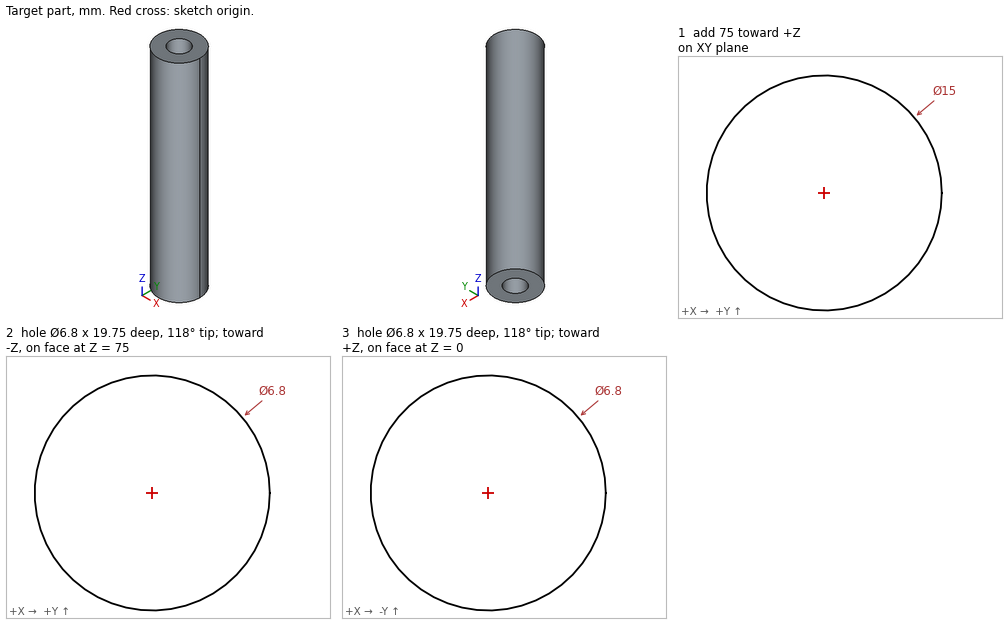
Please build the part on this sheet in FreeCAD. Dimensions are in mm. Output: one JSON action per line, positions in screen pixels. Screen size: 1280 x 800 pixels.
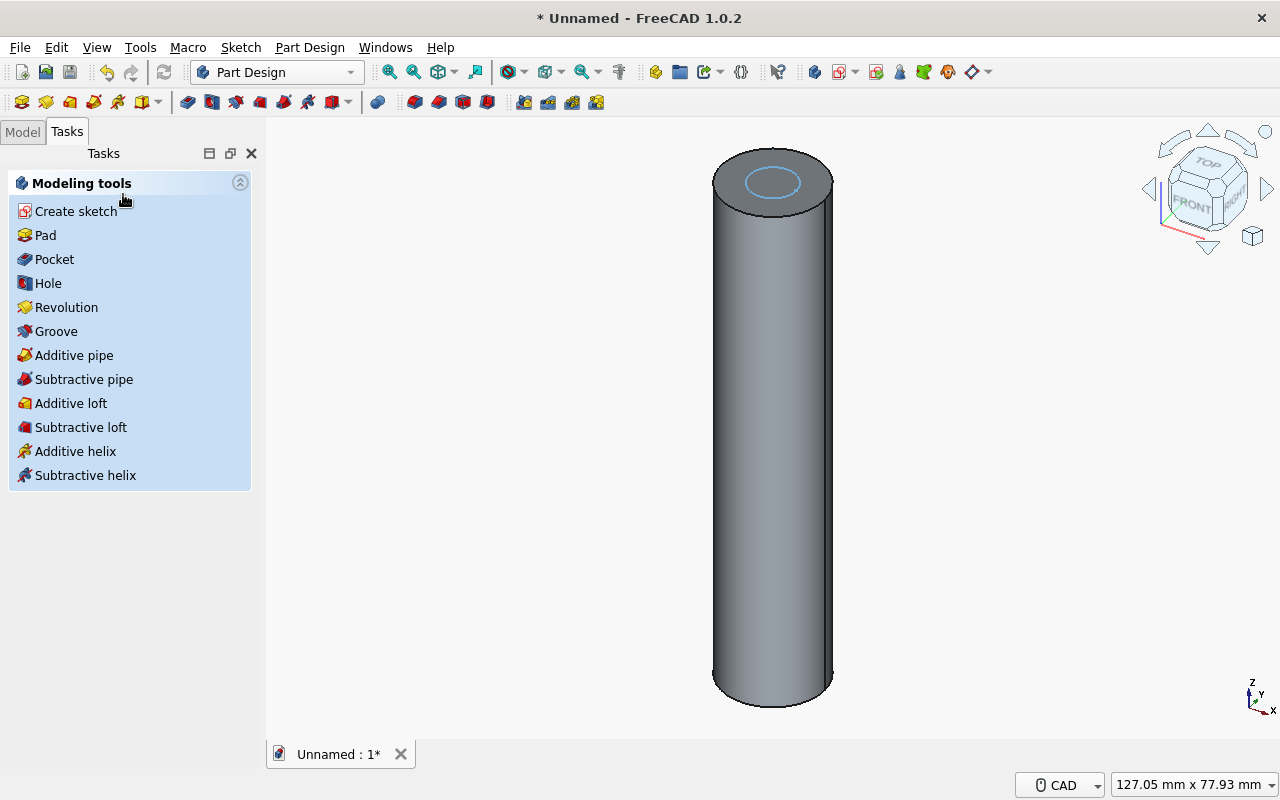
{"action": "left_click", "coordinate": [212, 102]}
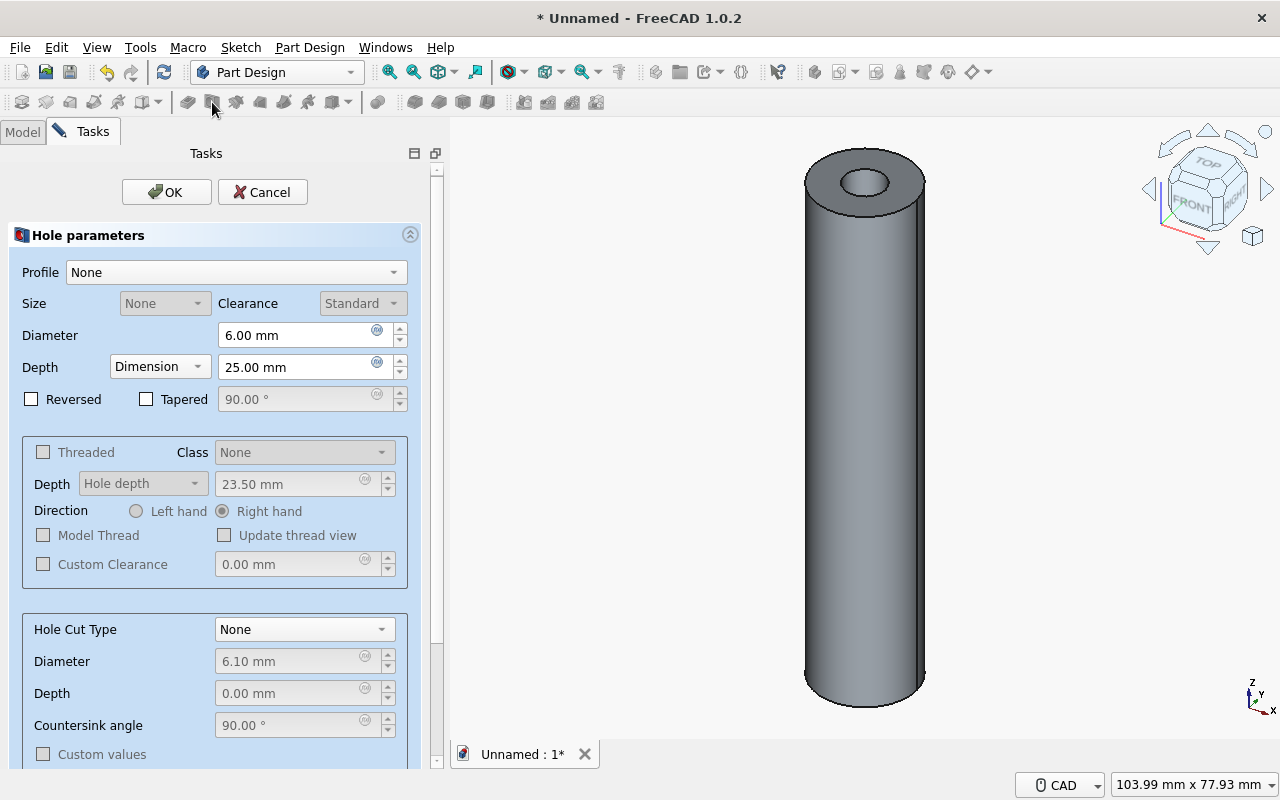
{"action": "triple_click", "coordinate": [305, 335]}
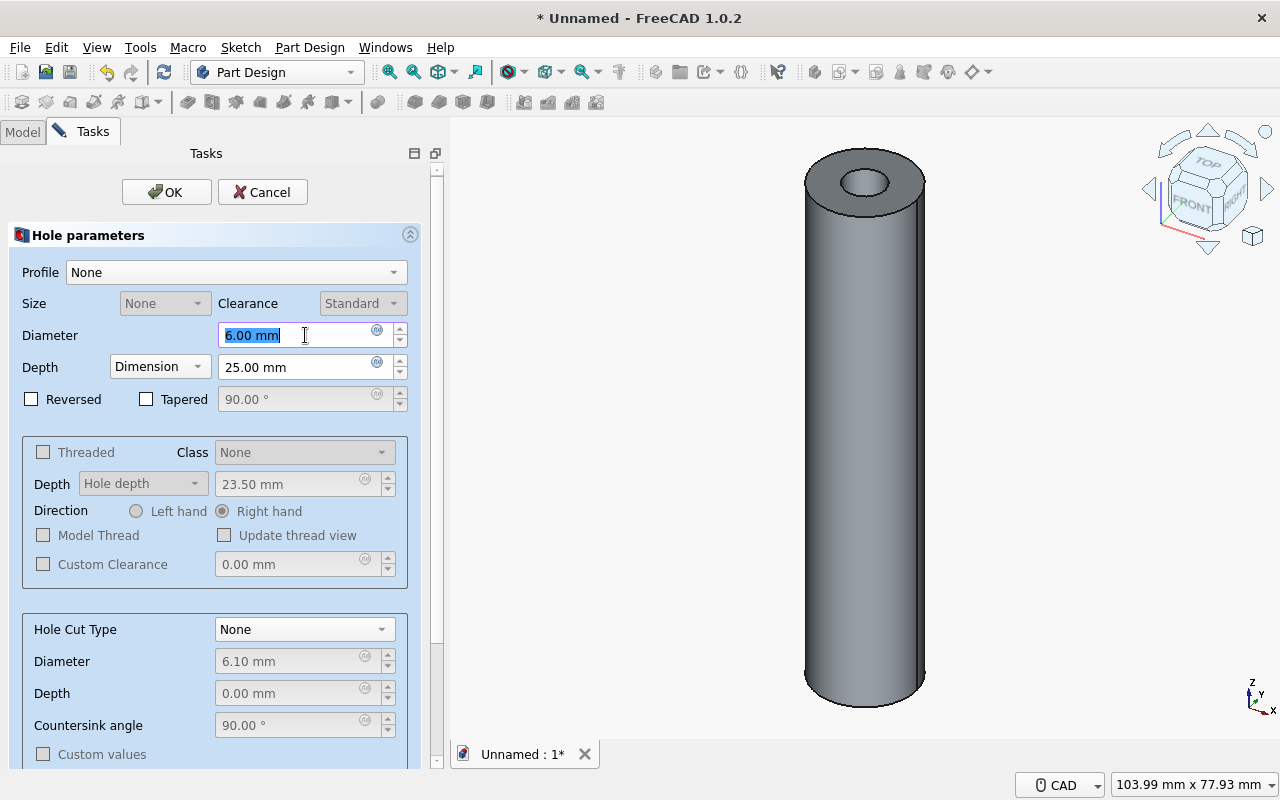
{"action": "type", "text": "6.8"}
{"action": "key", "text": "Tab"}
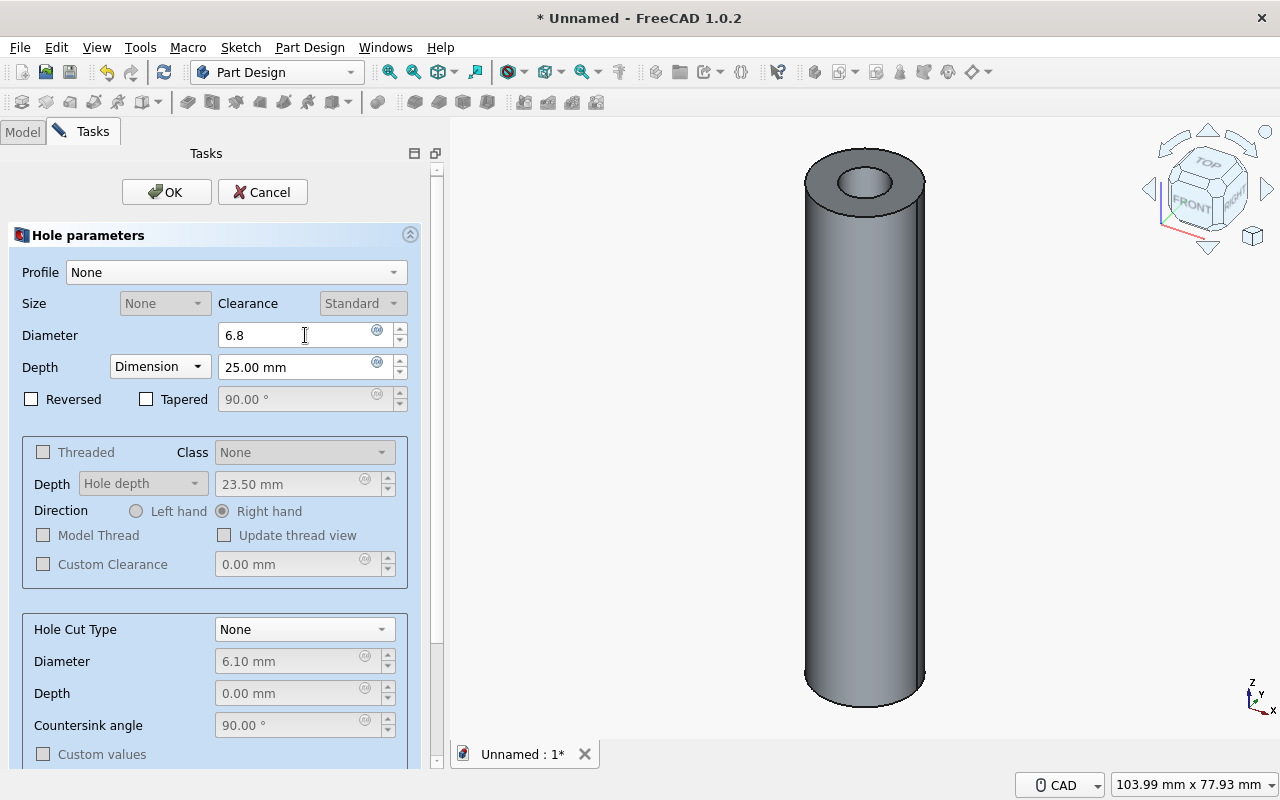
{"action": "triple_click", "coordinate": [305, 367]}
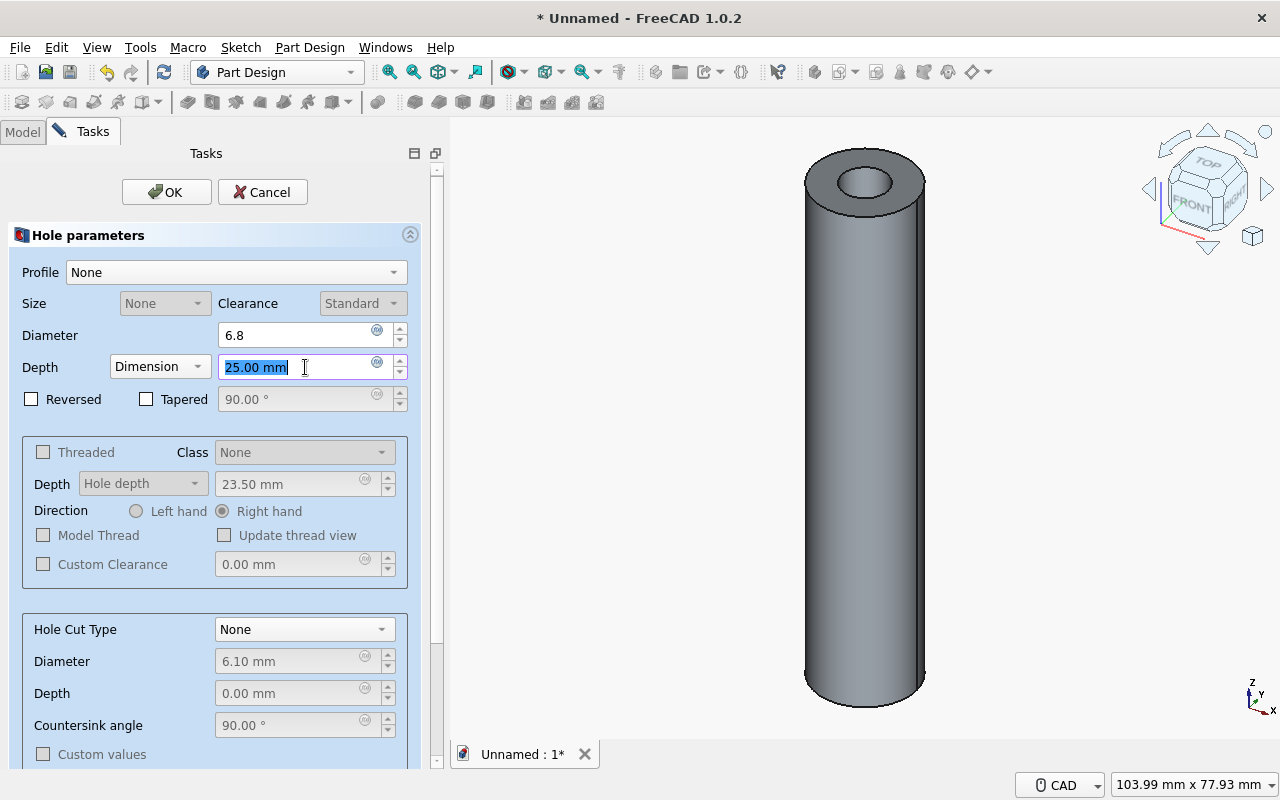
{"action": "type", "text": "19.75"}
{"action": "key", "text": "Tab"}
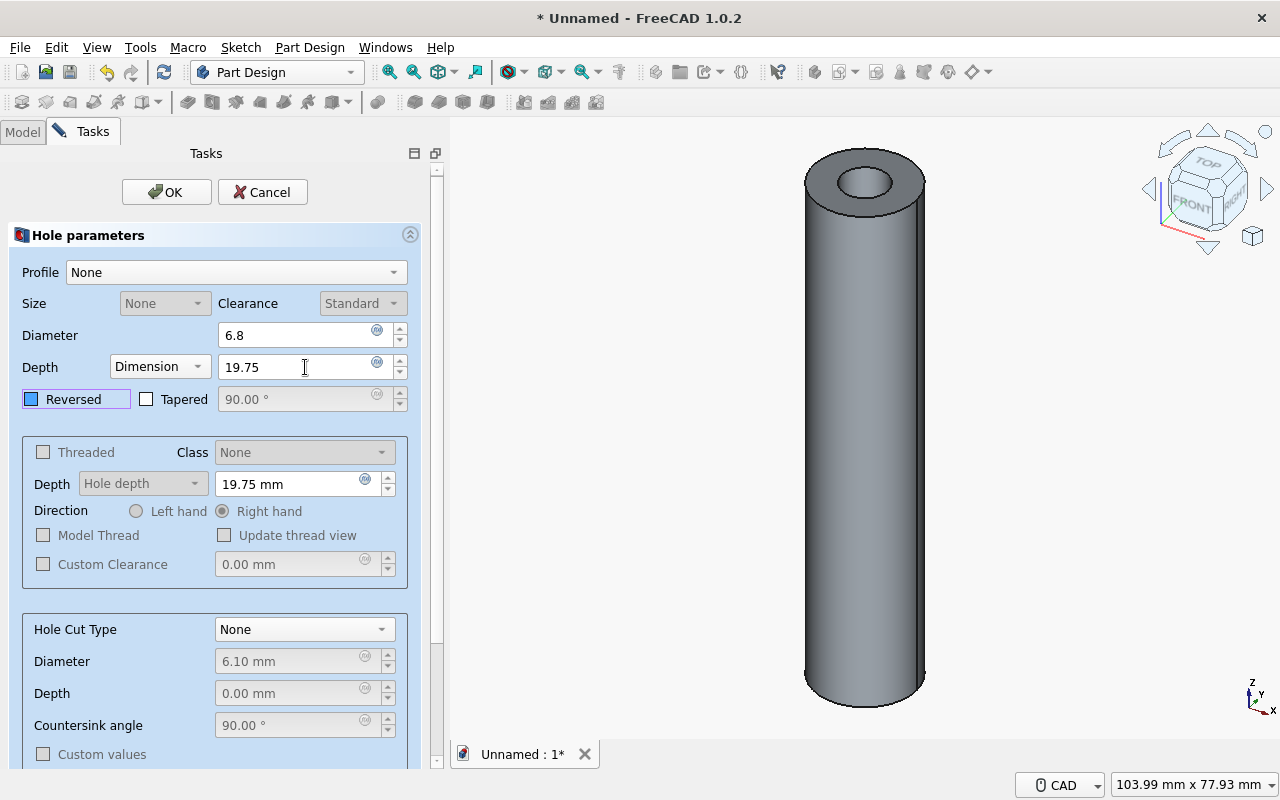
{"action": "left_click", "coordinate": [167, 192]}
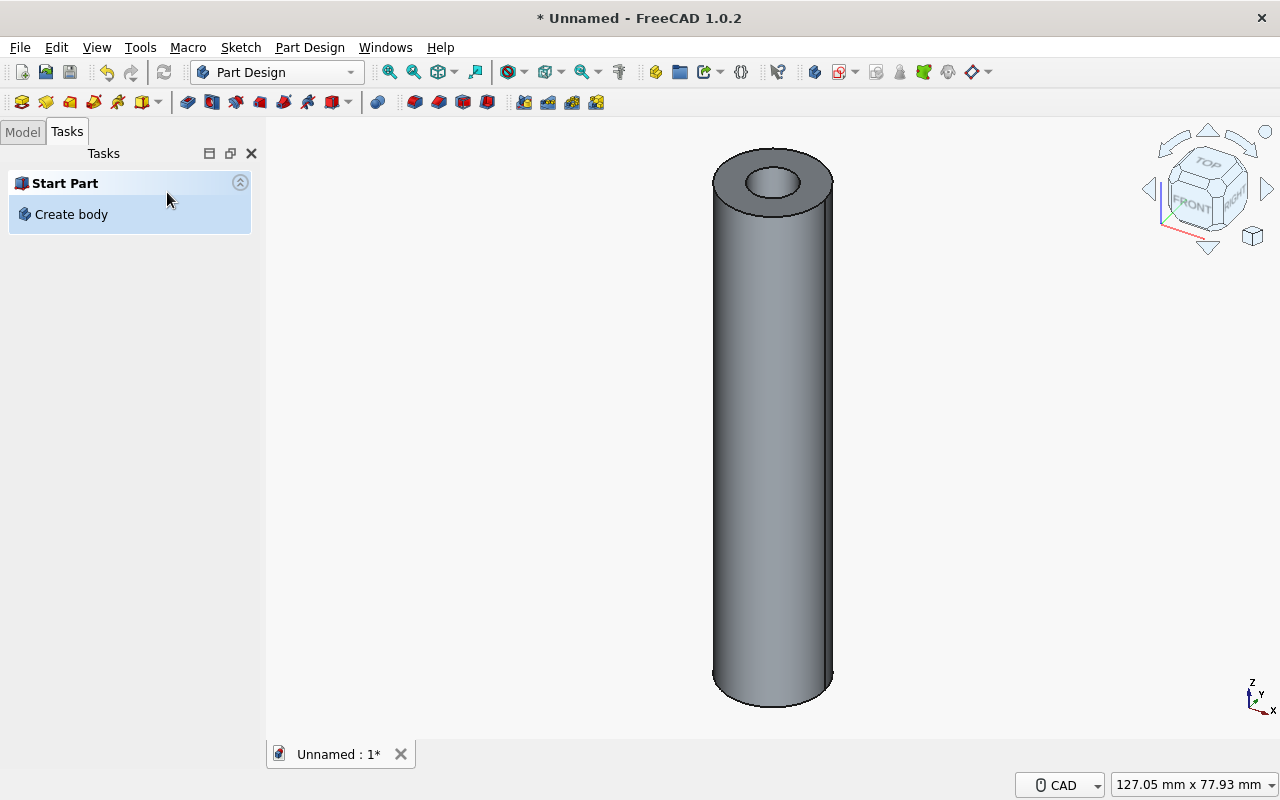
{"action": "key", "text": "5"}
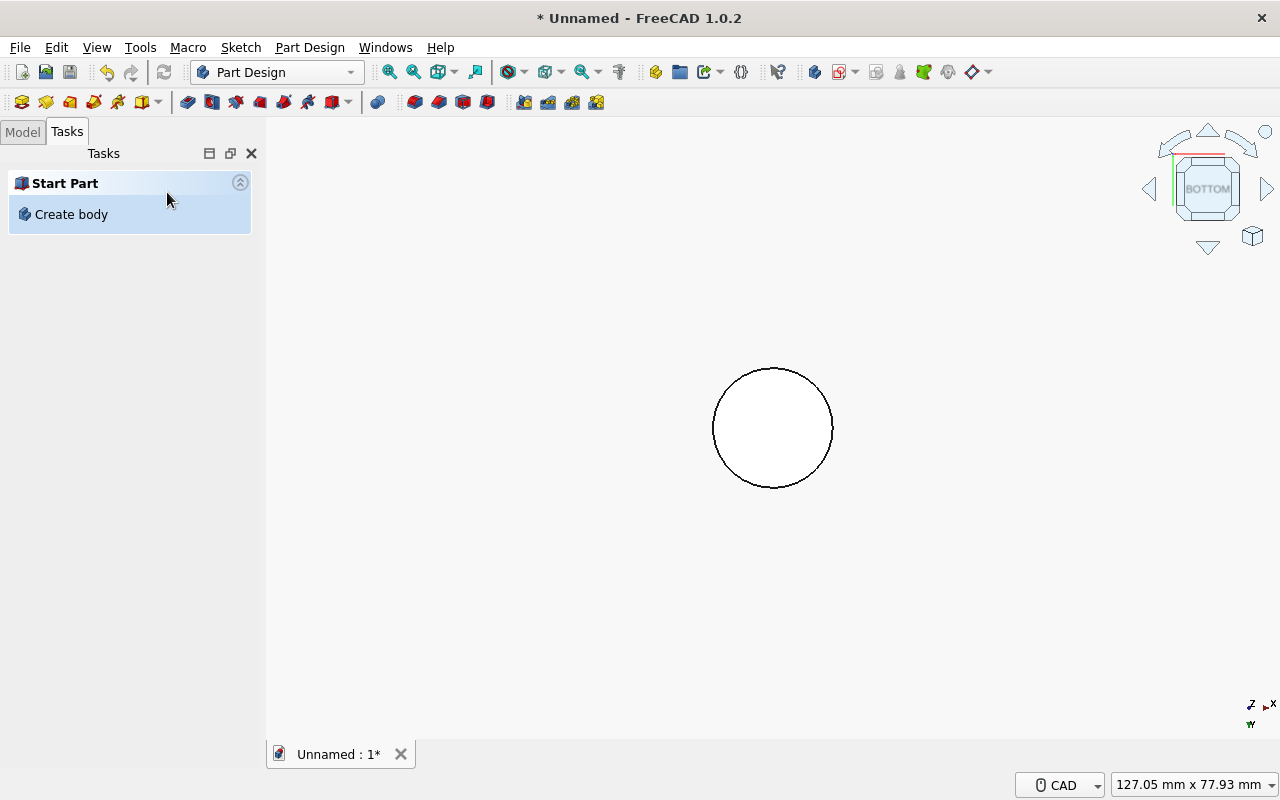
{"action": "left_click", "coordinate": [390, 72]}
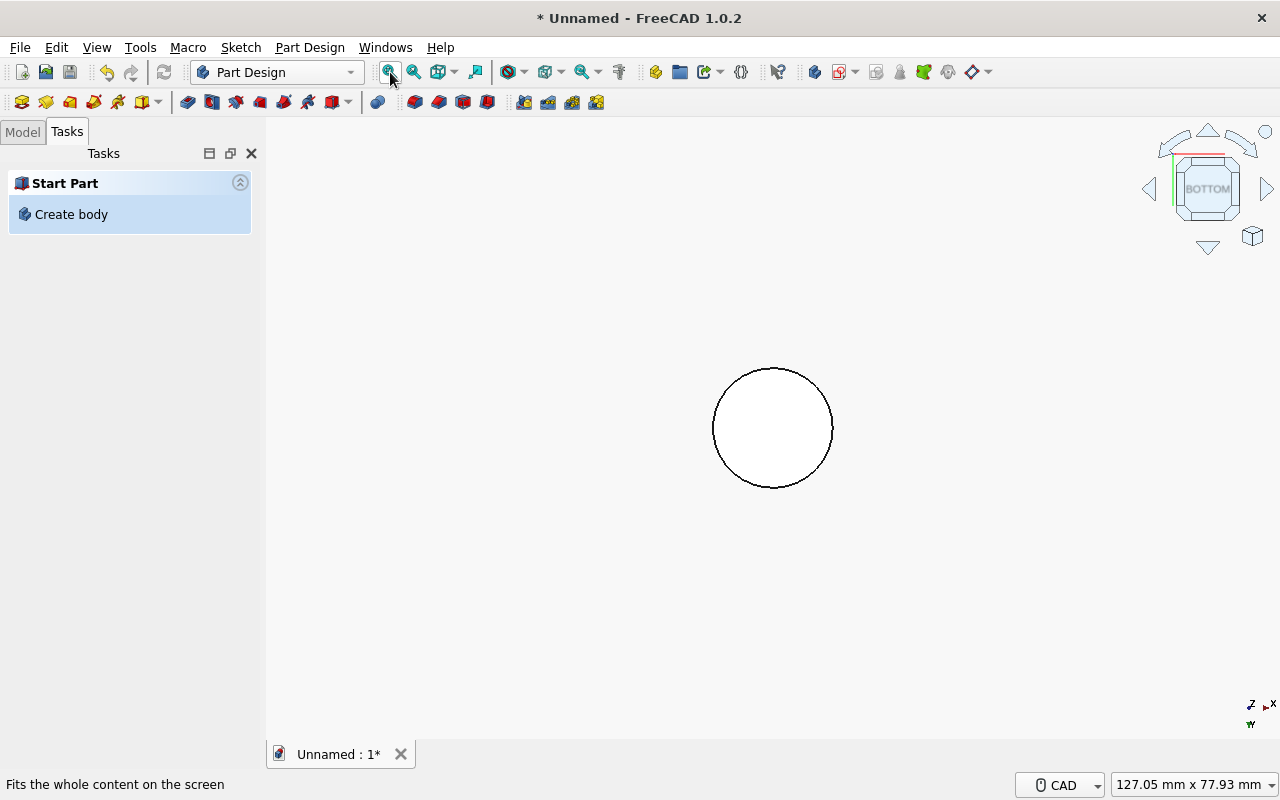
{"action": "left_click", "coordinate": [773, 427]}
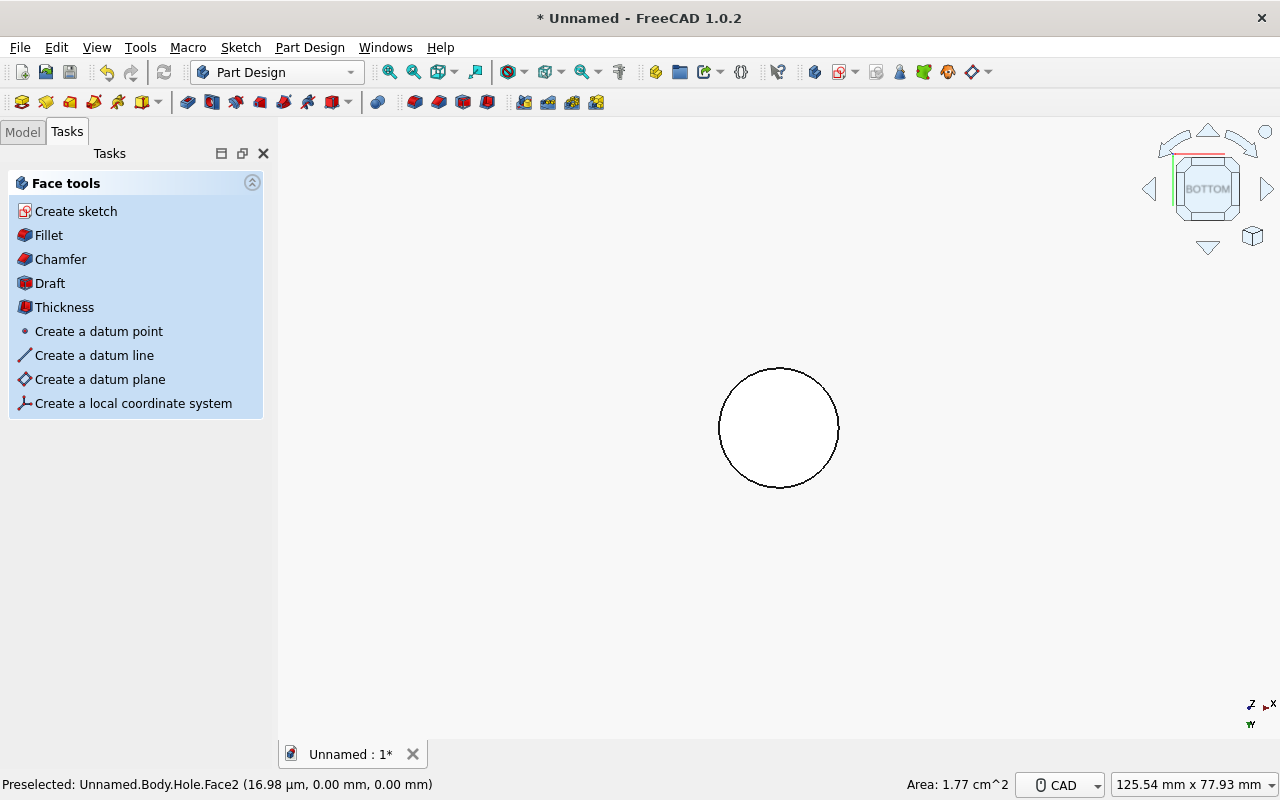
{"action": "left_click", "coordinate": [840, 72]}